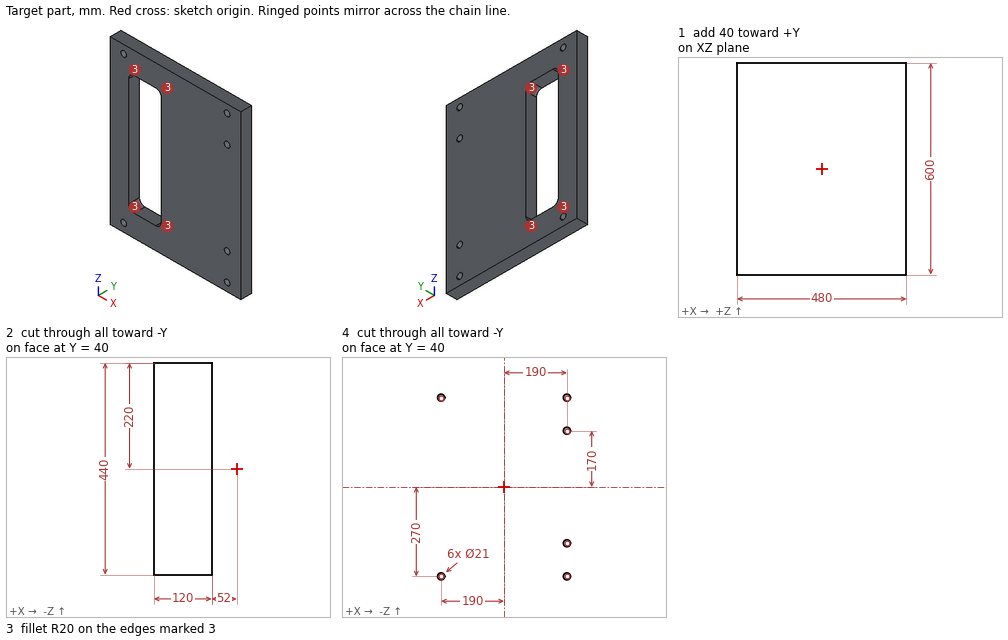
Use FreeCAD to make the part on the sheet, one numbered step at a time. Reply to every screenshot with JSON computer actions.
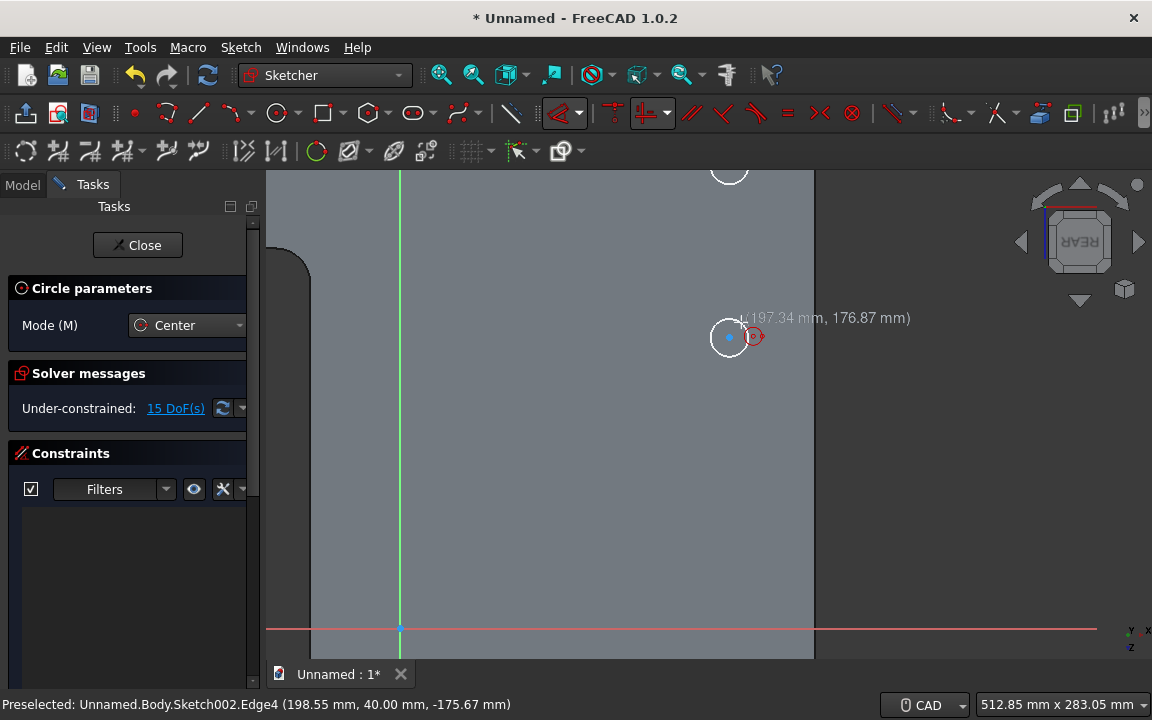
{"action": "scroll", "coordinate": [744, 322], "scroll_direction": "down", "scroll_amount": 6}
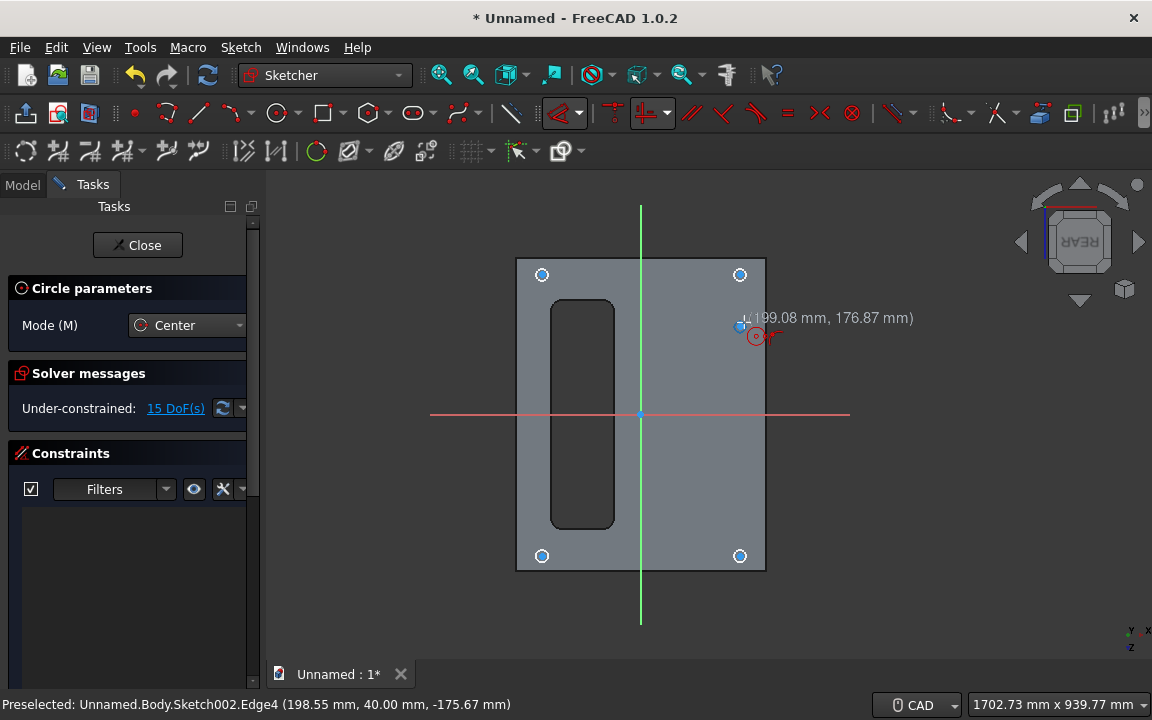
{"action": "scroll", "coordinate": [740, 503], "scroll_direction": "up", "scroll_amount": 8}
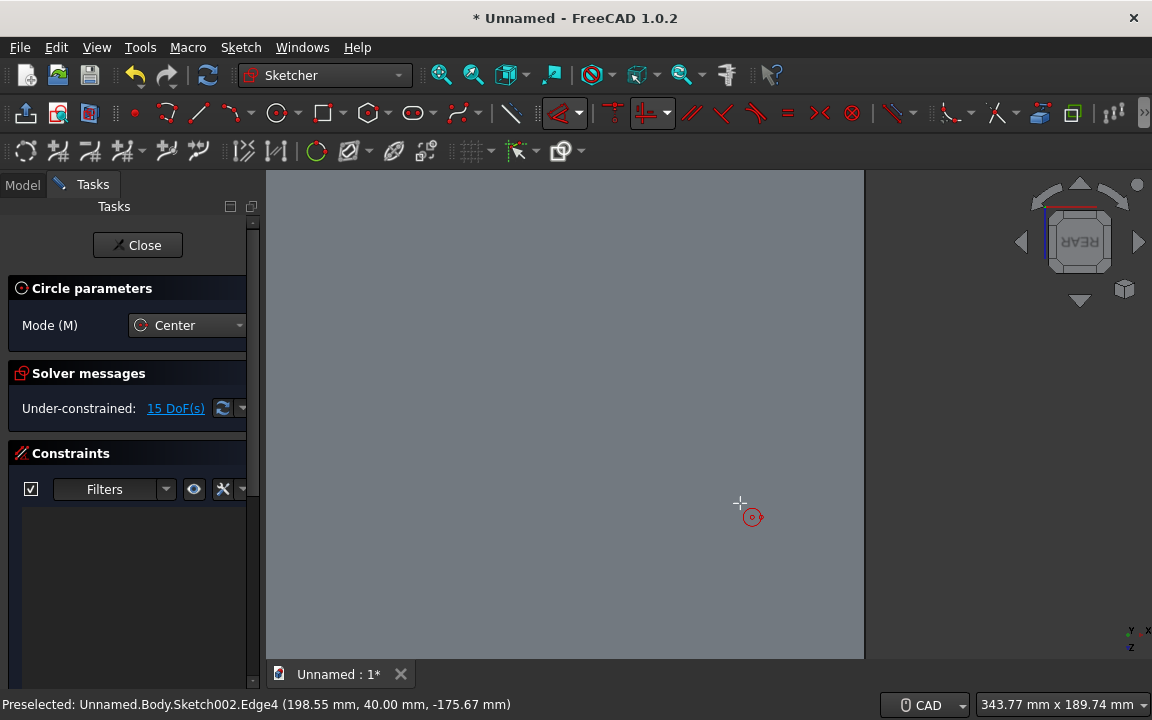
{"action": "scroll", "coordinate": [740, 504], "scroll_direction": "down", "scroll_amount": 8}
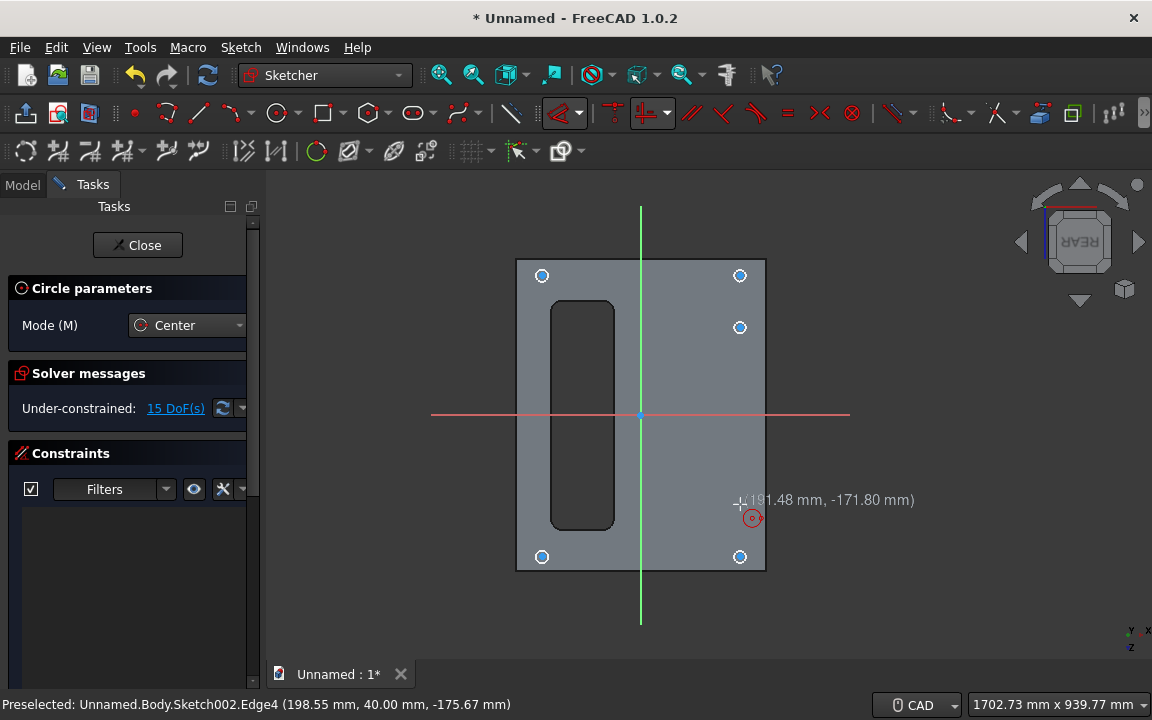
{"action": "left_click", "coordinate": [740, 504]}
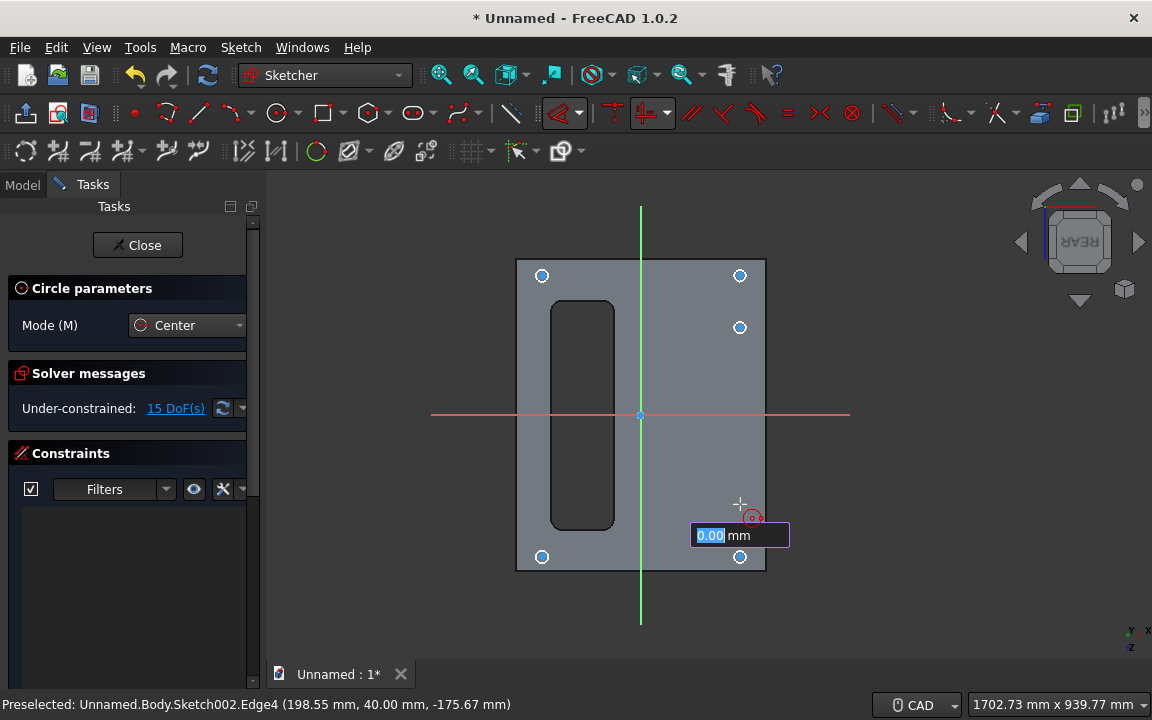
{"action": "scroll", "coordinate": [744, 500], "scroll_direction": "up", "scroll_amount": 6}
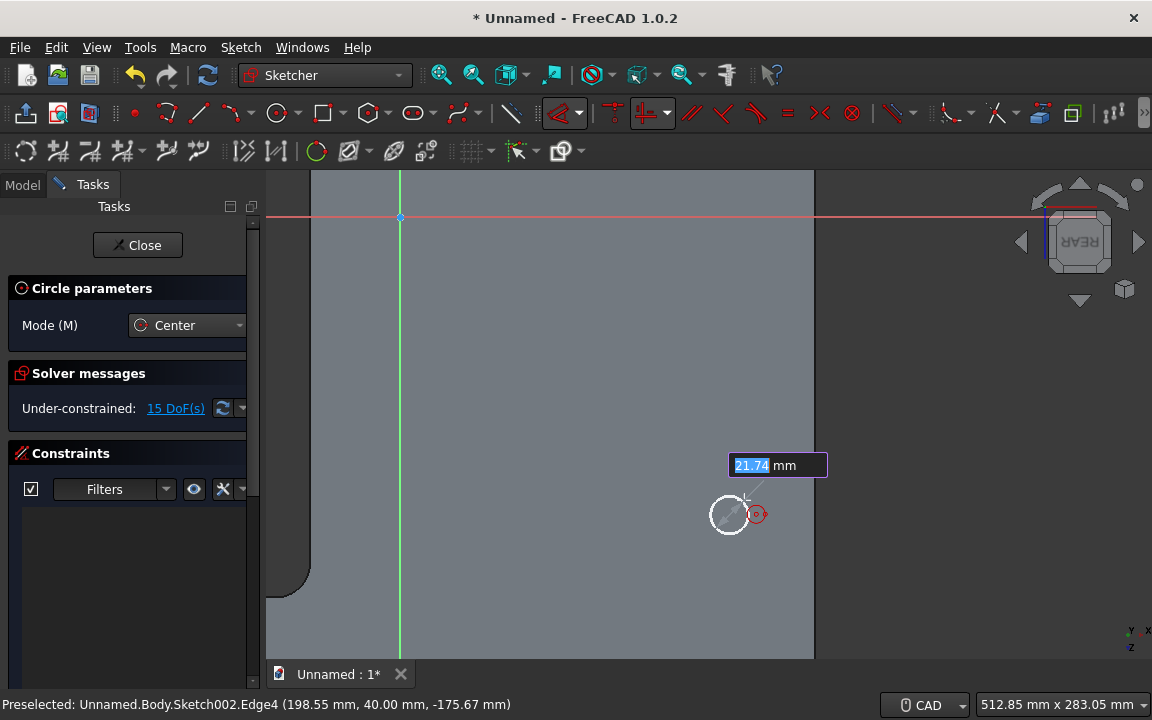
{"action": "left_click", "coordinate": [741, 498]}
{"action": "key", "text": "Escape"}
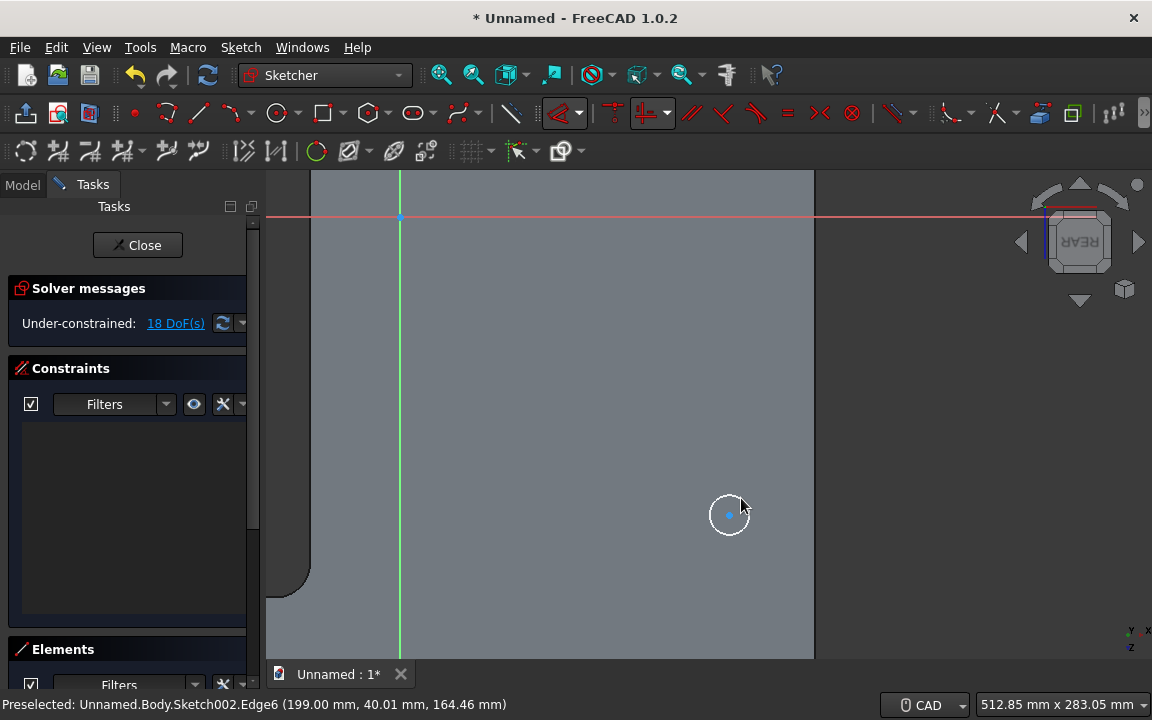
{"action": "scroll", "coordinate": [744, 499], "scroll_direction": "down", "scroll_amount": 6}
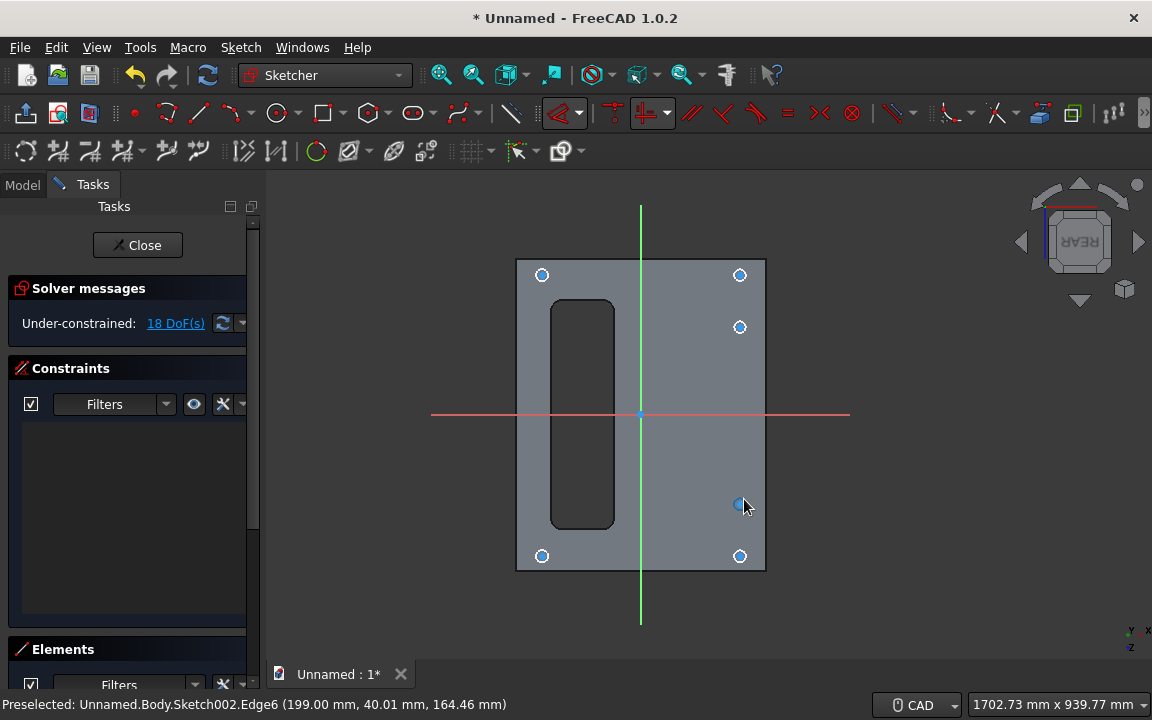
{"action": "scroll", "coordinate": [546, 552], "scroll_direction": "up", "scroll_amount": 5}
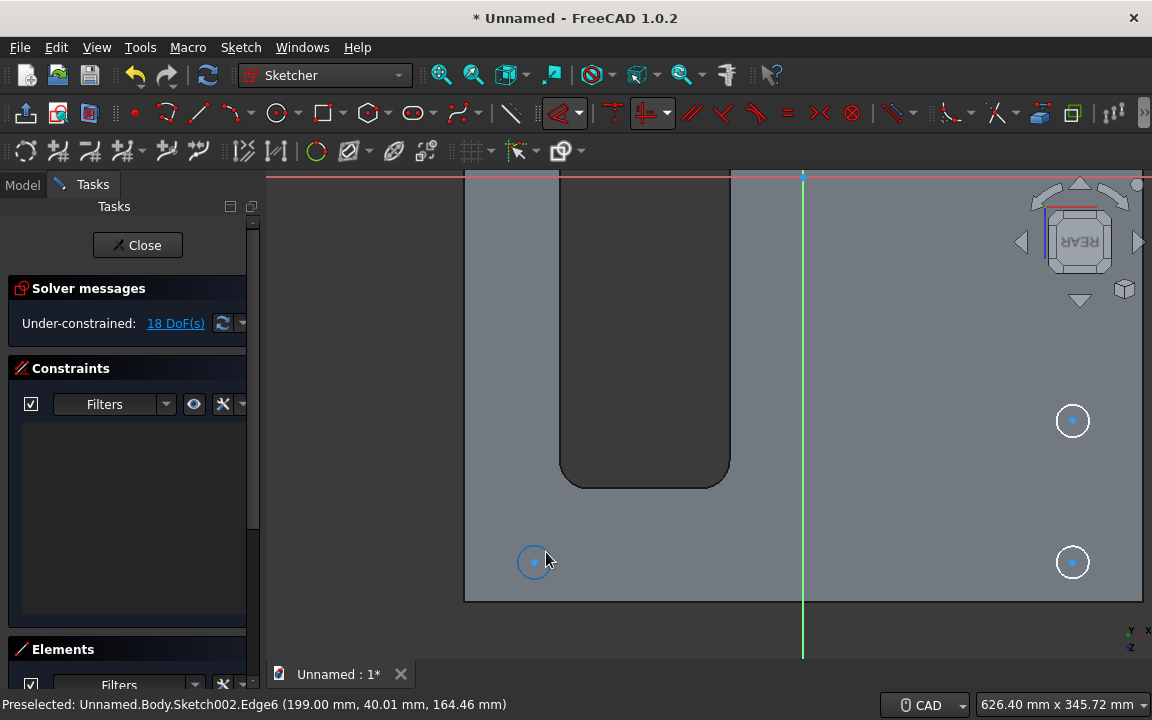
{"action": "left_click", "coordinate": [546, 550]}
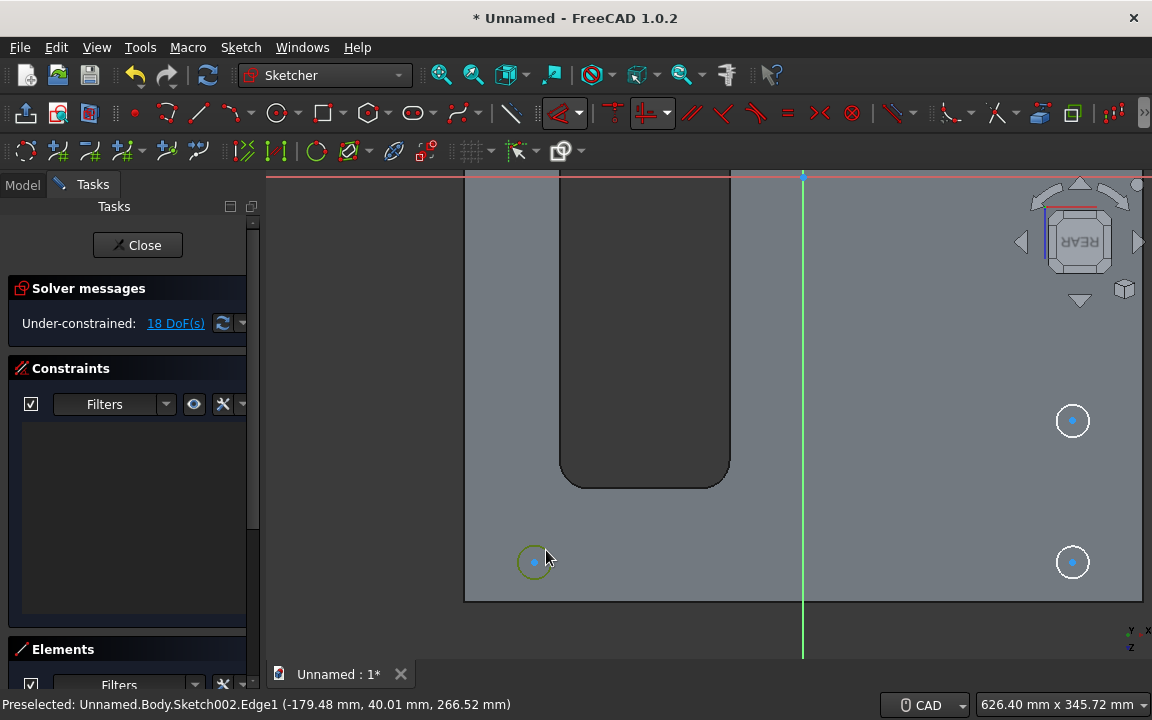
{"action": "scroll", "coordinate": [546, 553], "scroll_direction": "down", "scroll_amount": 5}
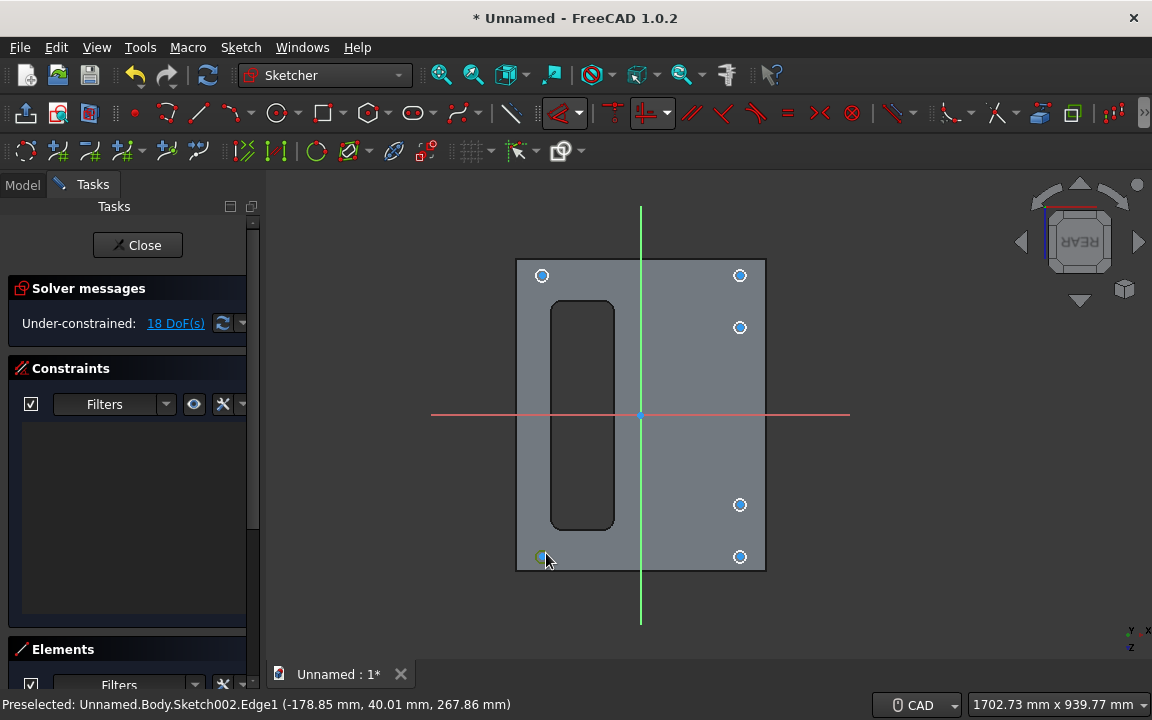
{"action": "scroll", "coordinate": [546, 271], "scroll_direction": "up", "scroll_amount": 5}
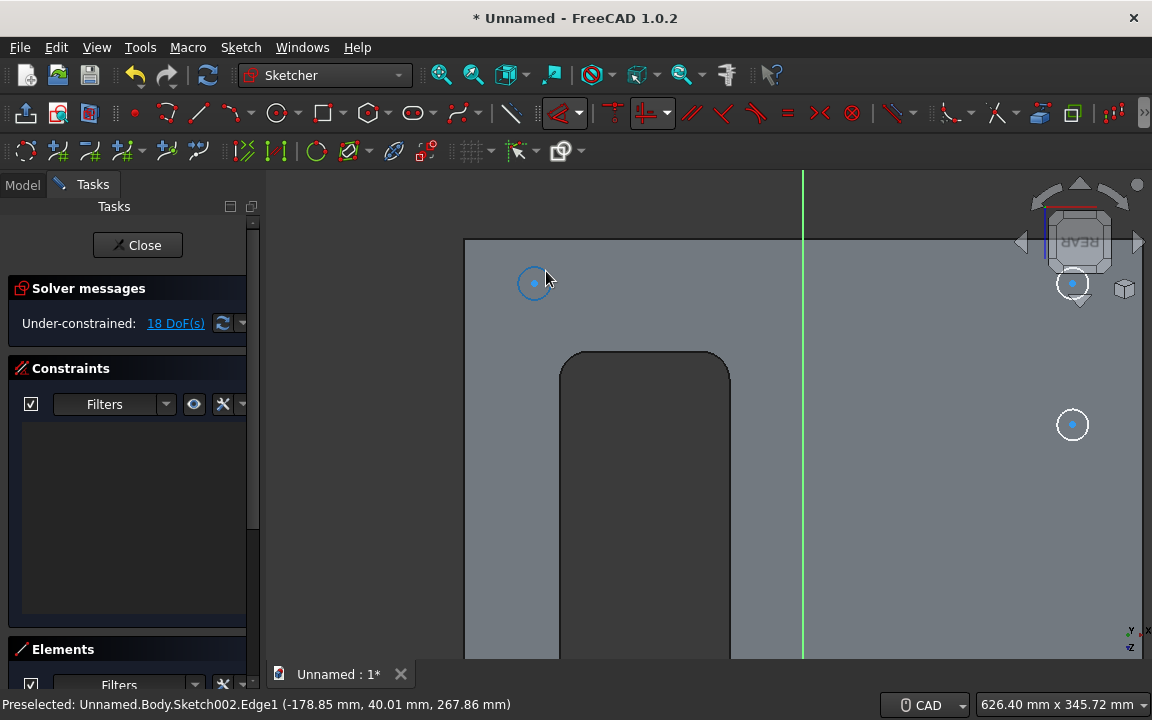
{"action": "left_click", "coordinate": [546, 272]}